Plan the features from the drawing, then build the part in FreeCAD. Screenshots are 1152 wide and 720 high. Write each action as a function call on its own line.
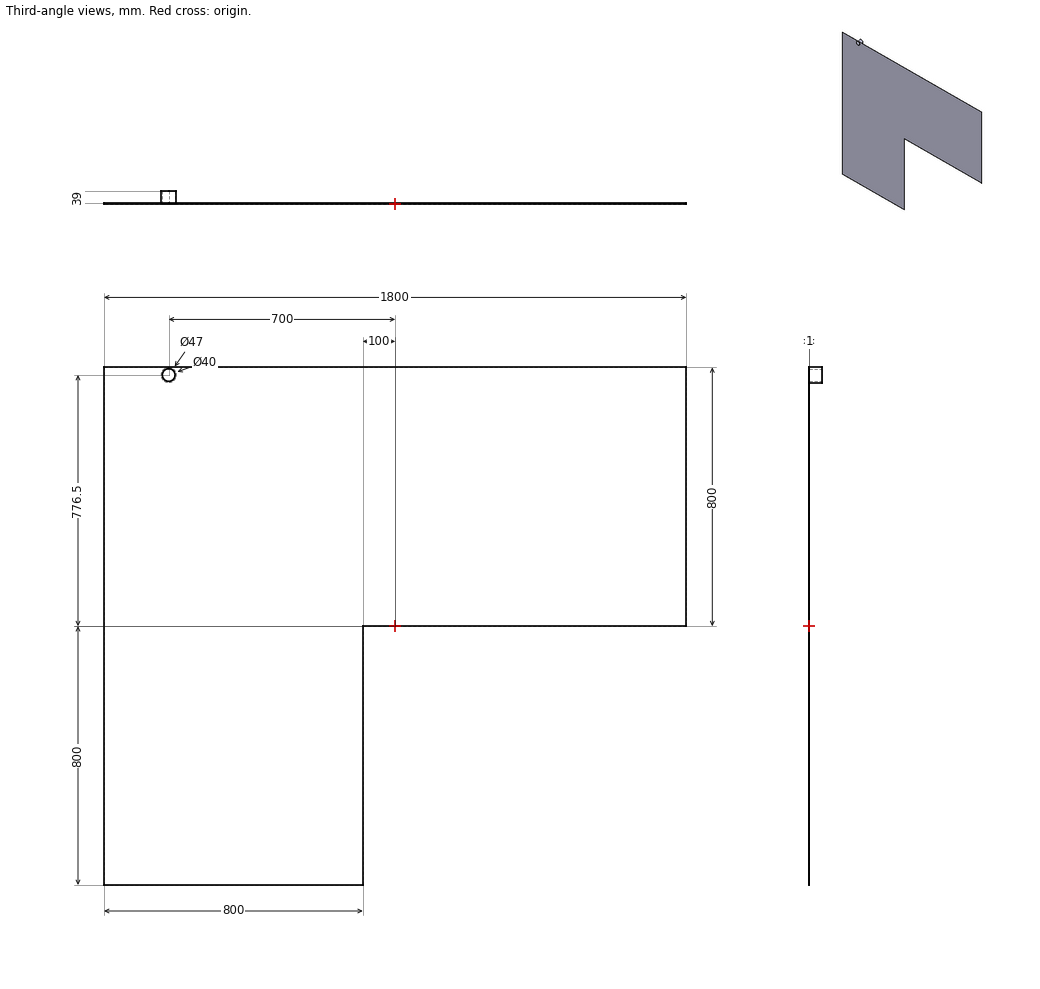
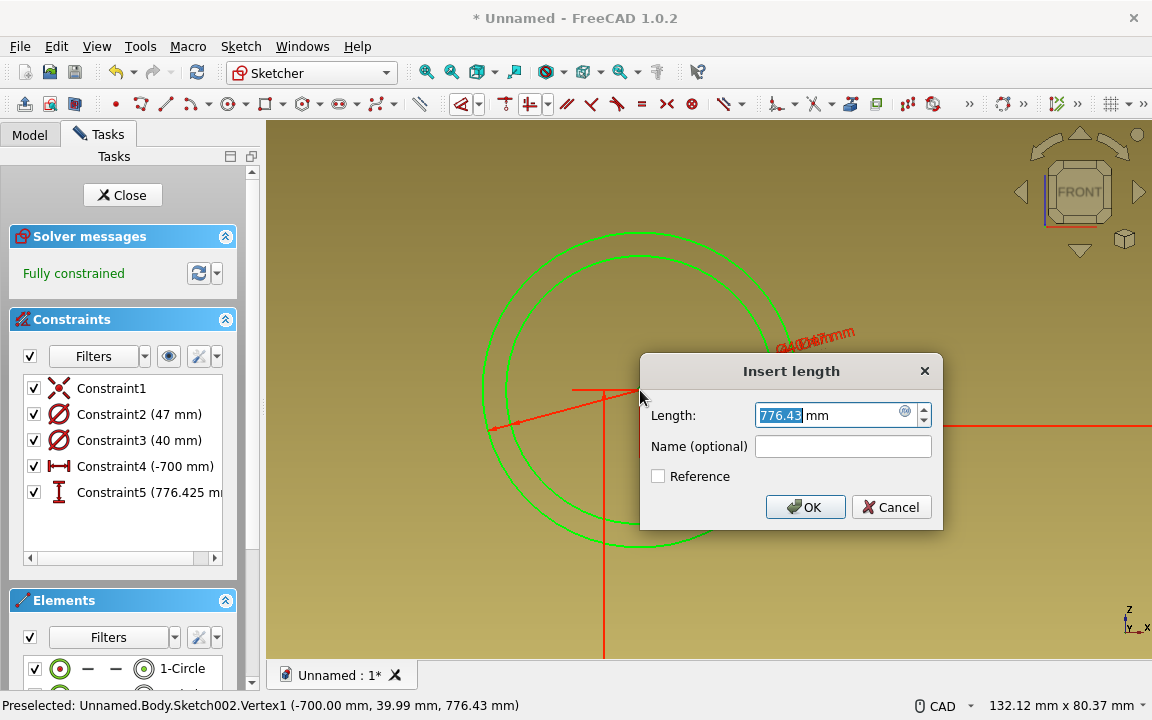
text(776.5)
key(Return)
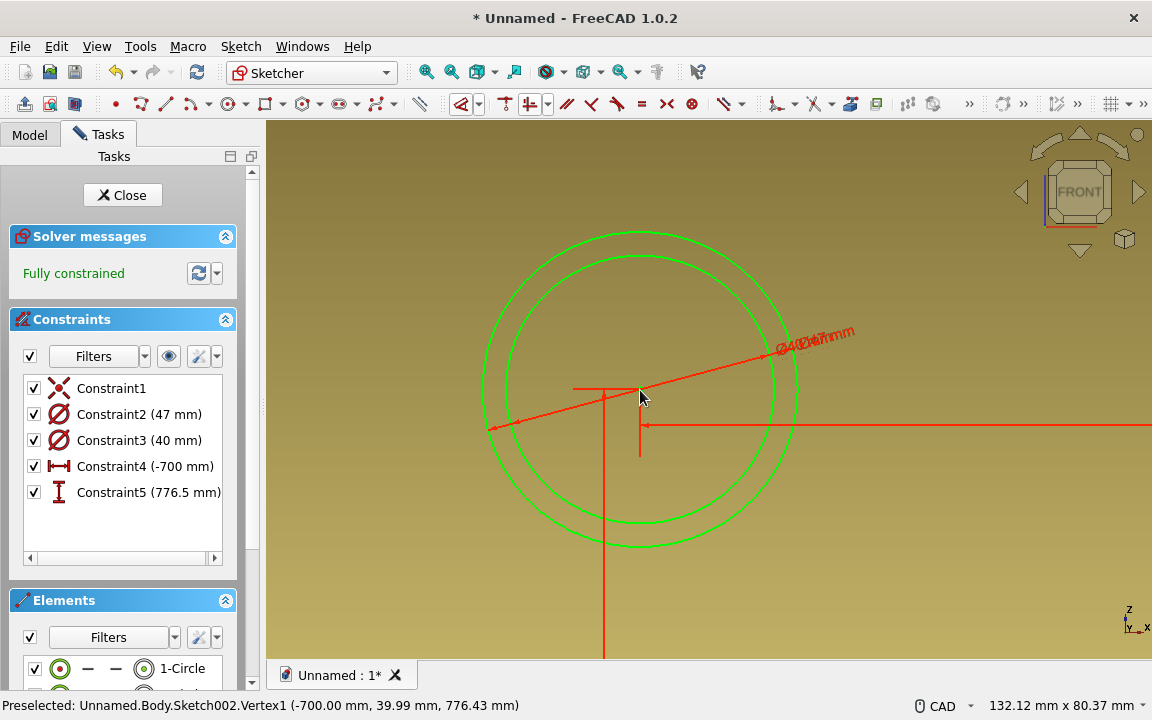
click(123, 195)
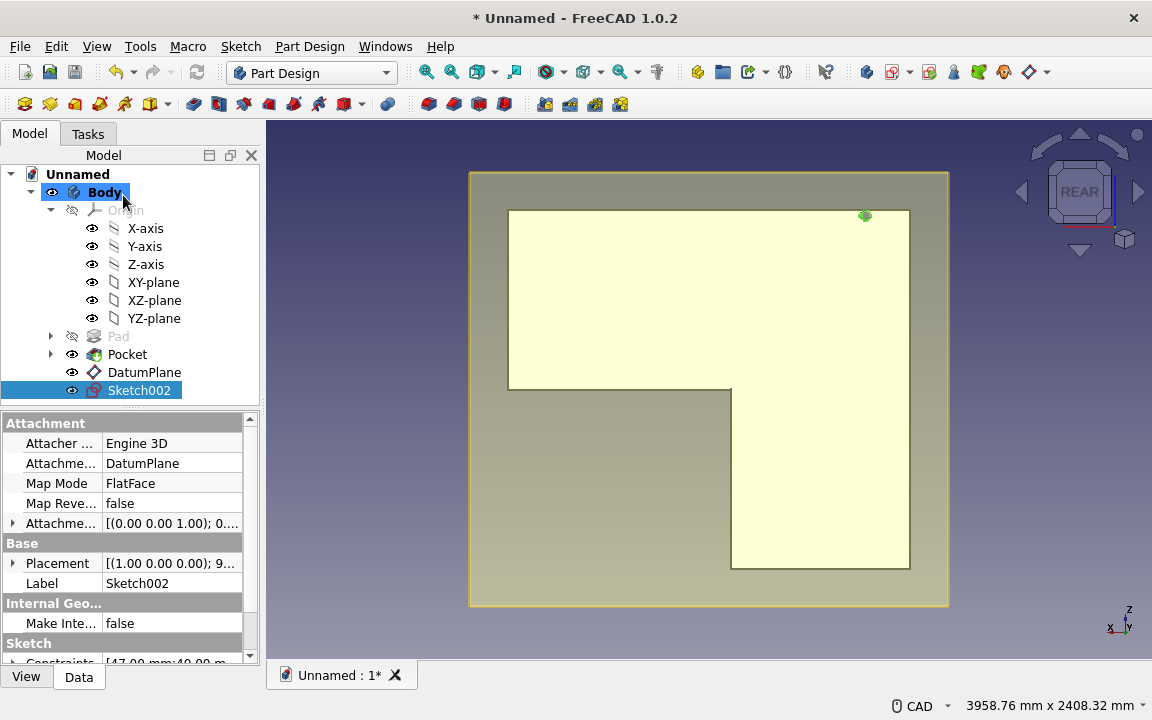
click(25, 104)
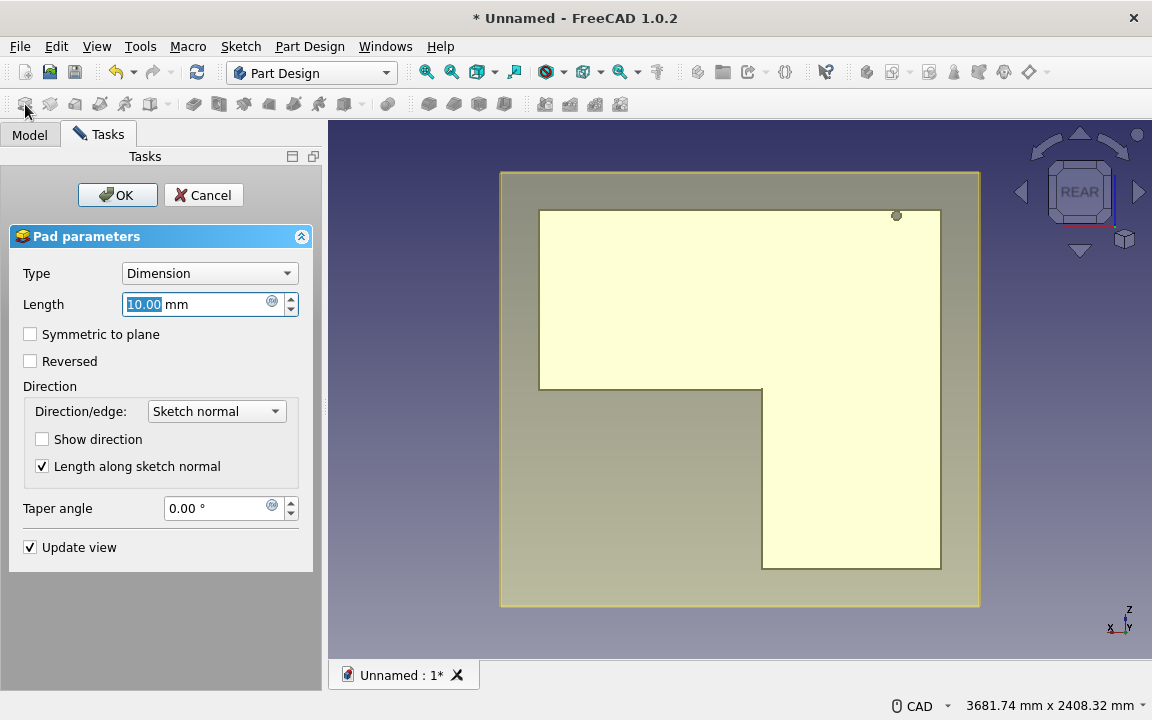
text(39)
key(Tab)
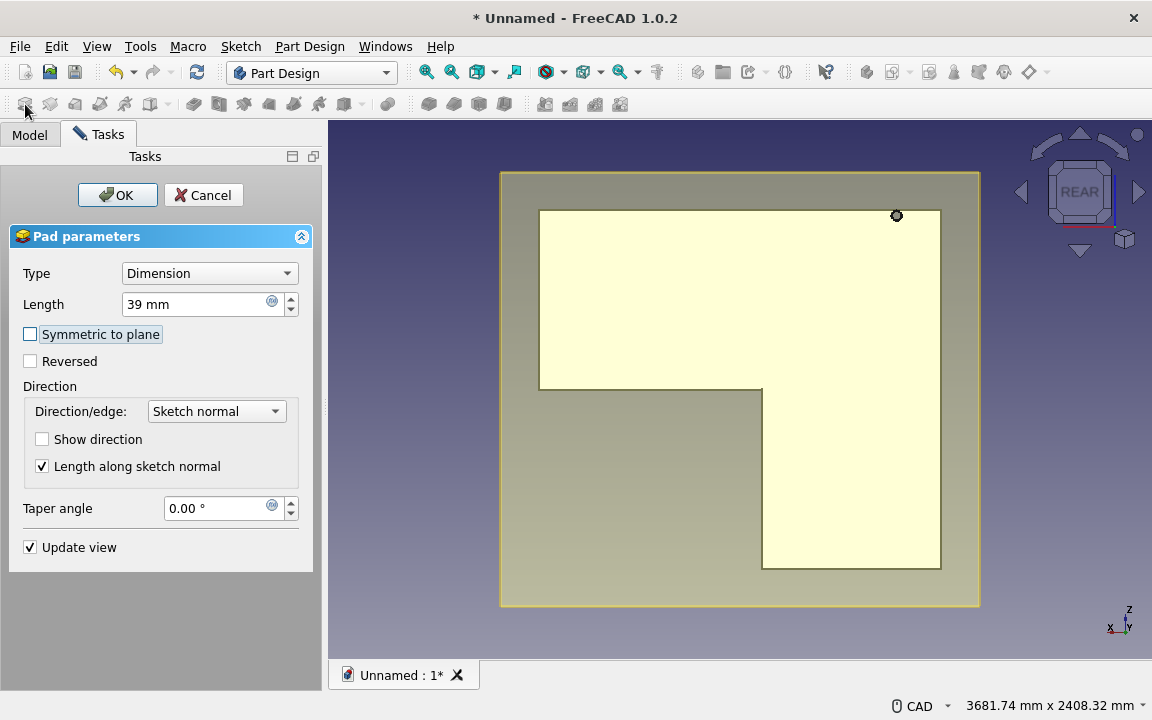
click(118, 195)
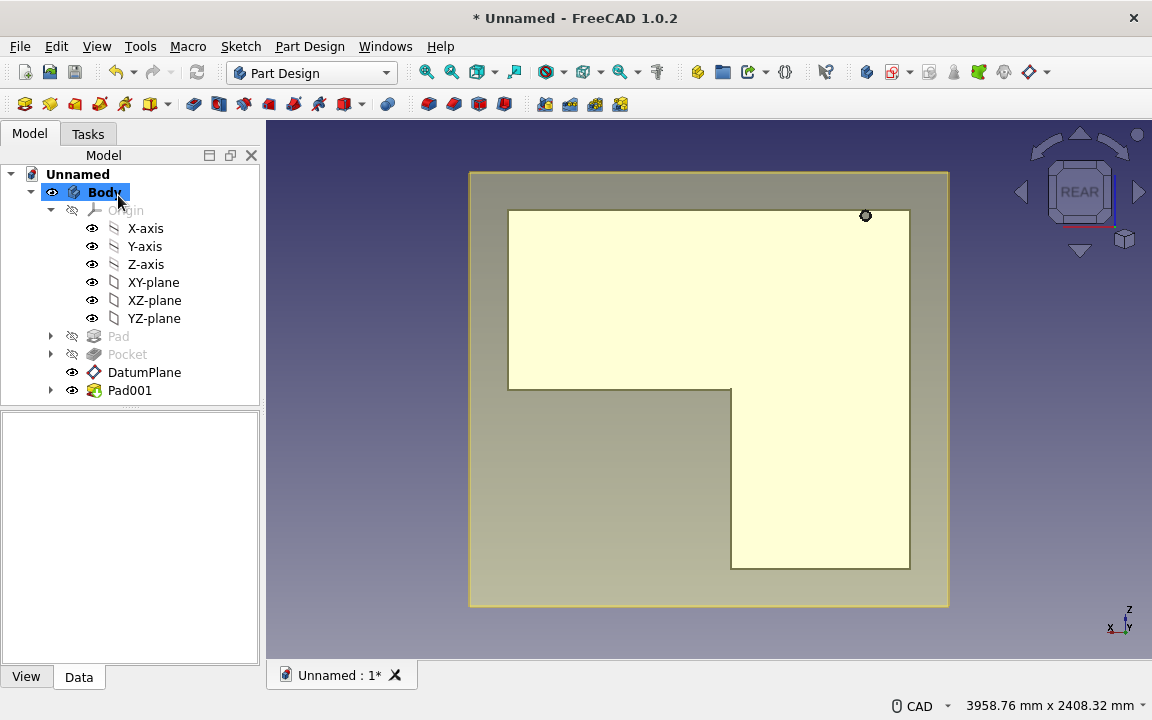
click(117, 372)
key(space)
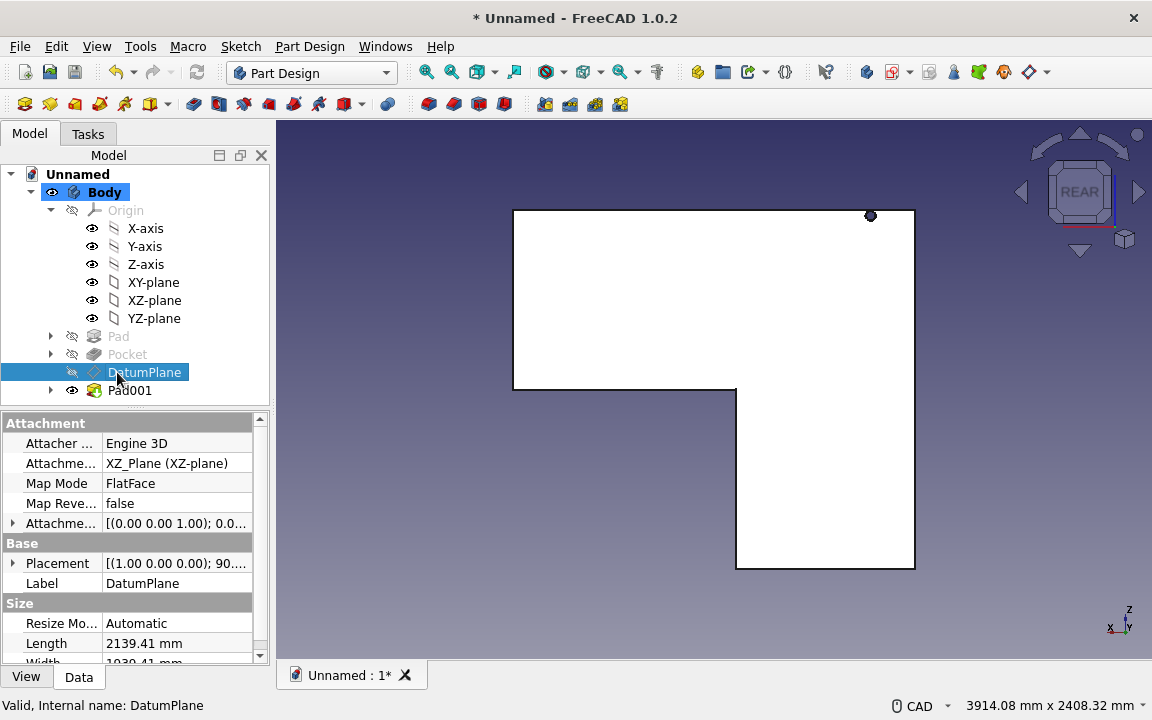
key(0)